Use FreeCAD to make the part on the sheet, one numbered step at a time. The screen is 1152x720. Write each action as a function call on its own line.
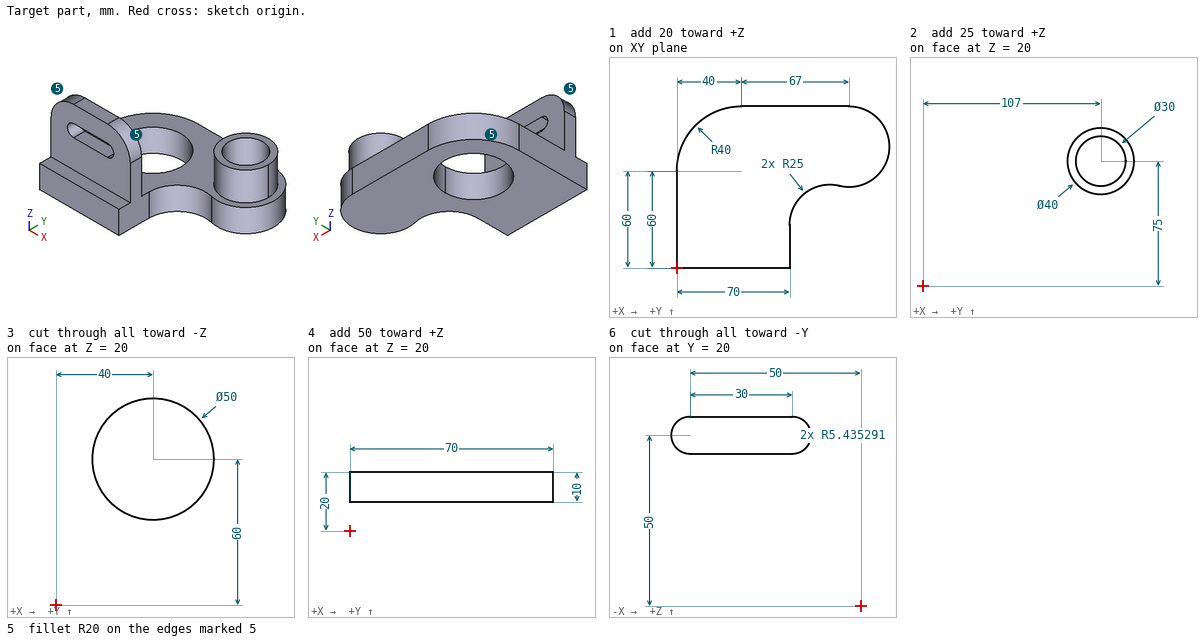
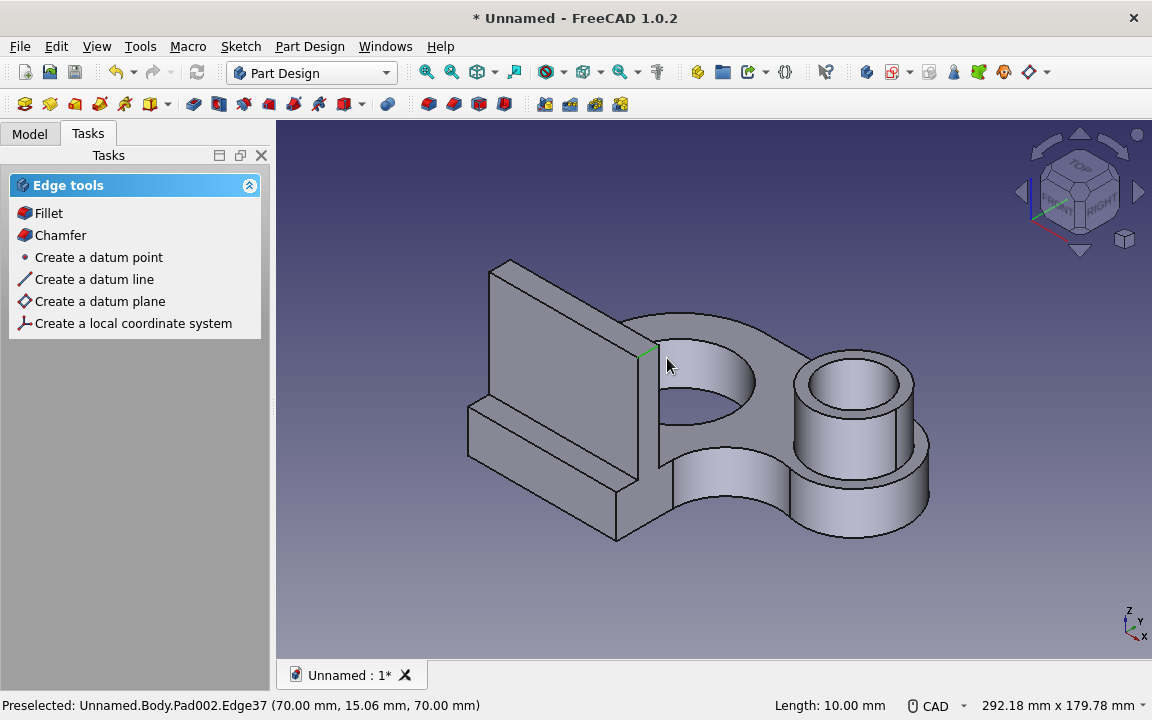
key(2)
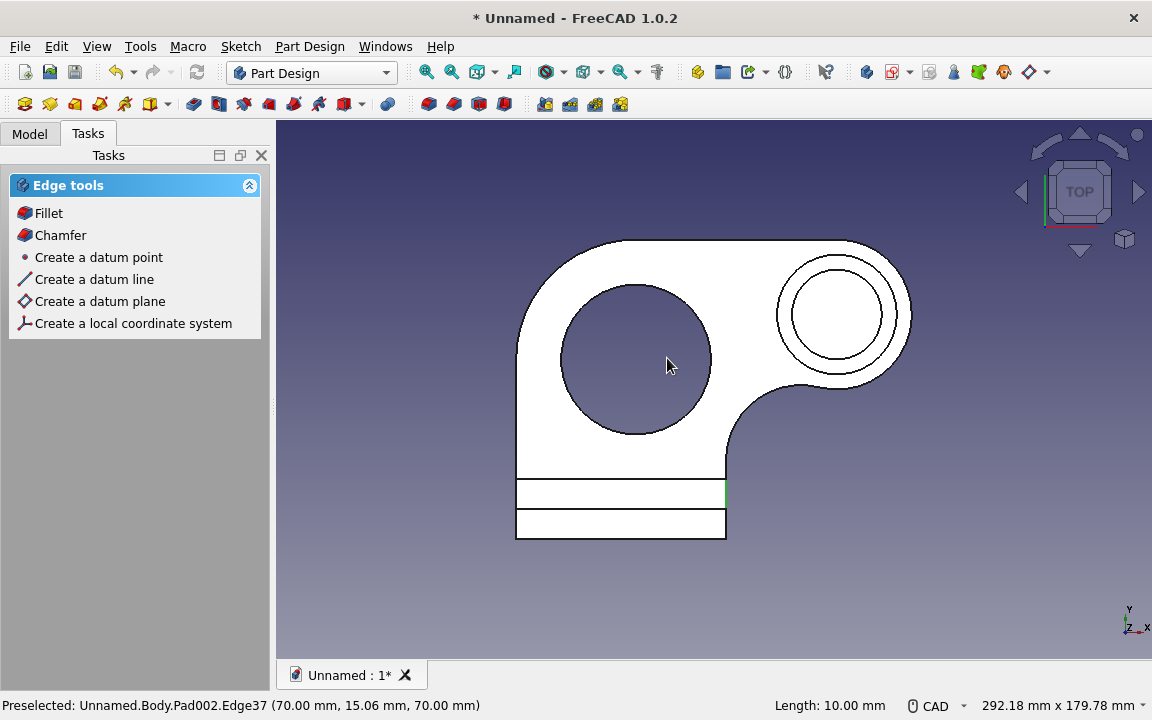
click(516, 493, ctrl)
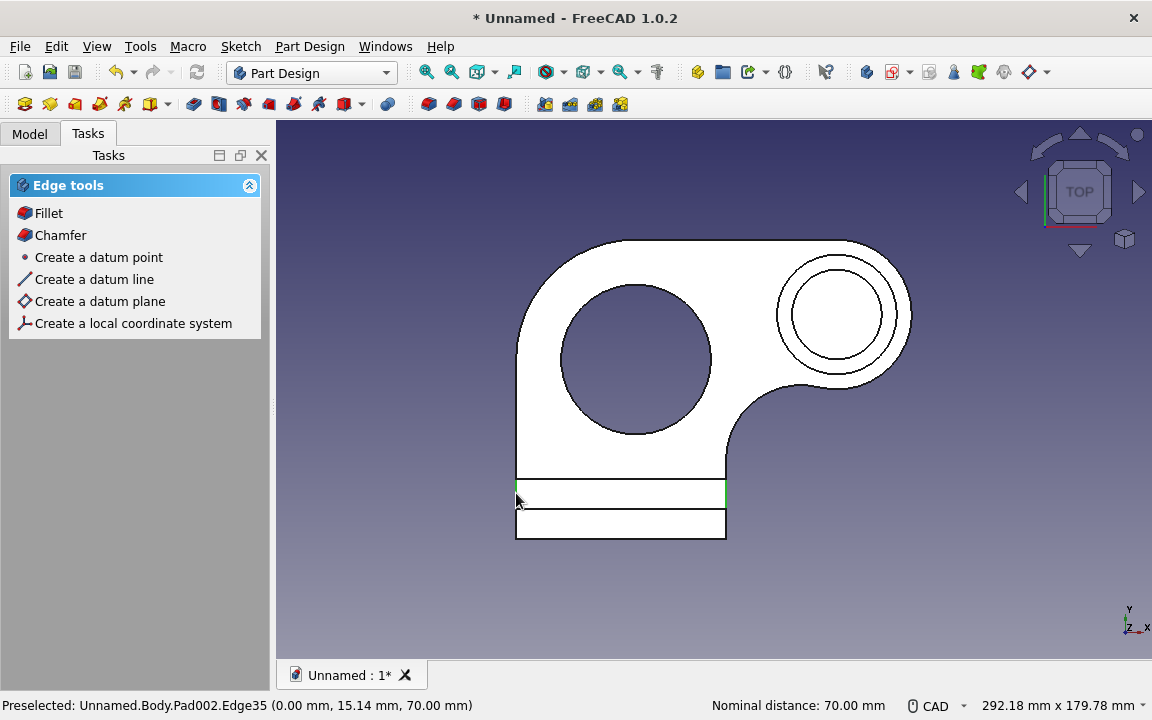
click(429, 104)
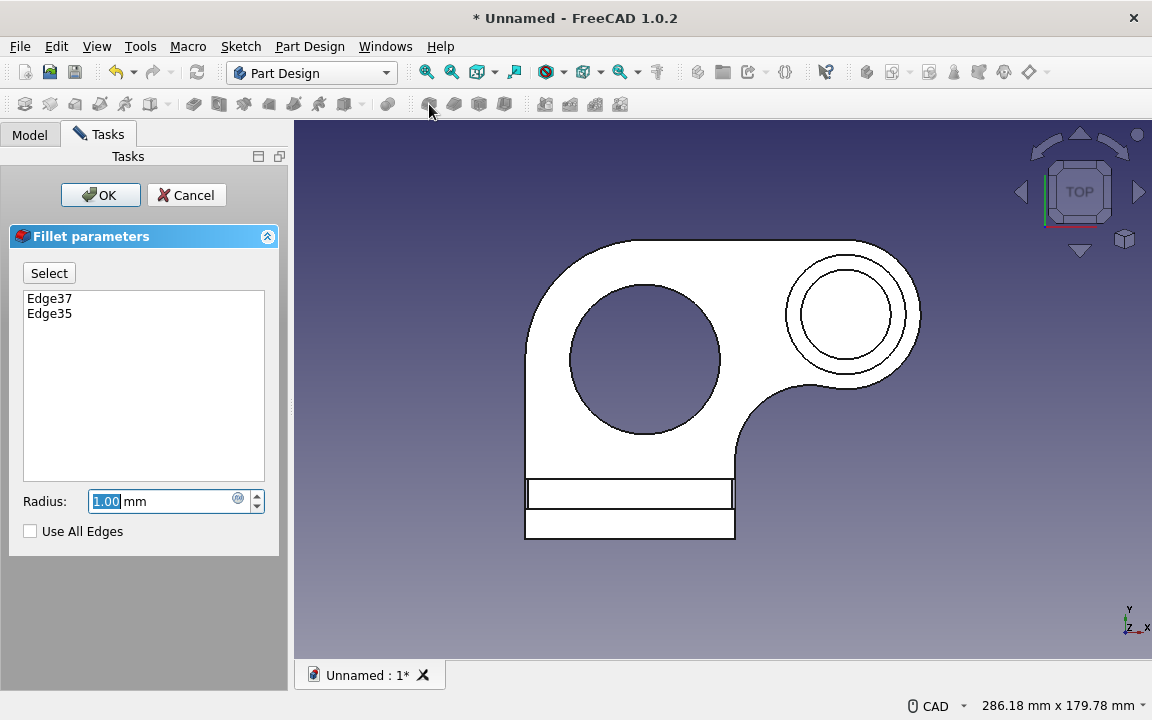
text(20)
key(Tab)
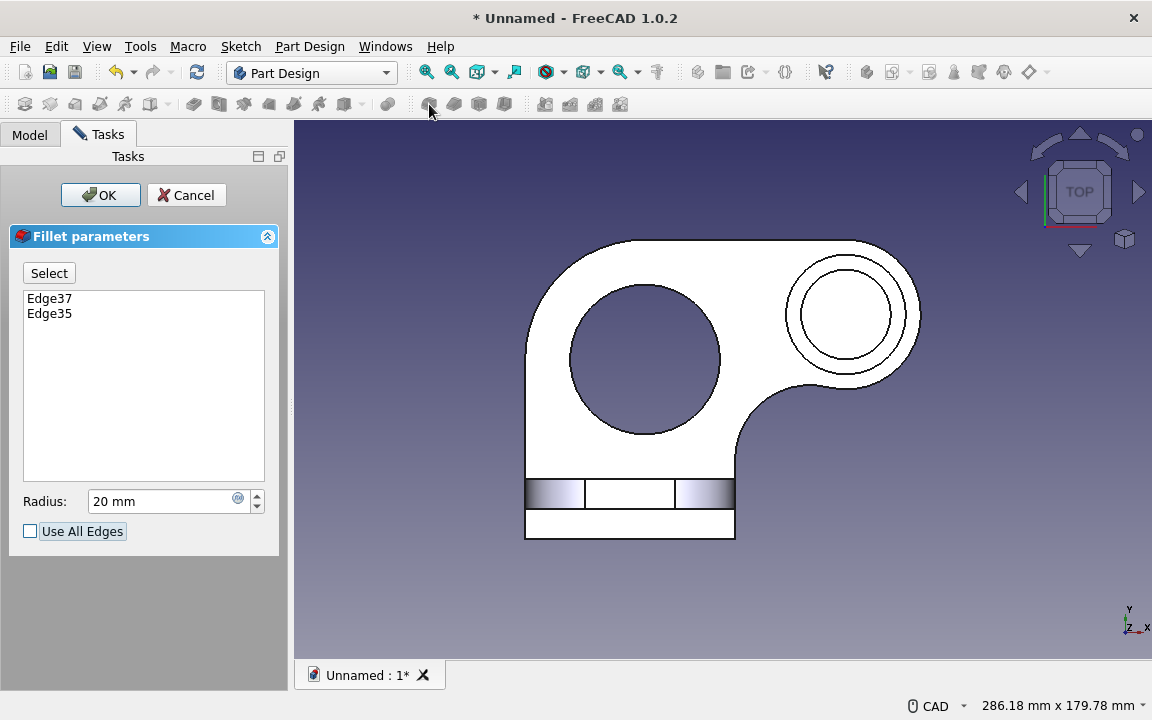
click(101, 195)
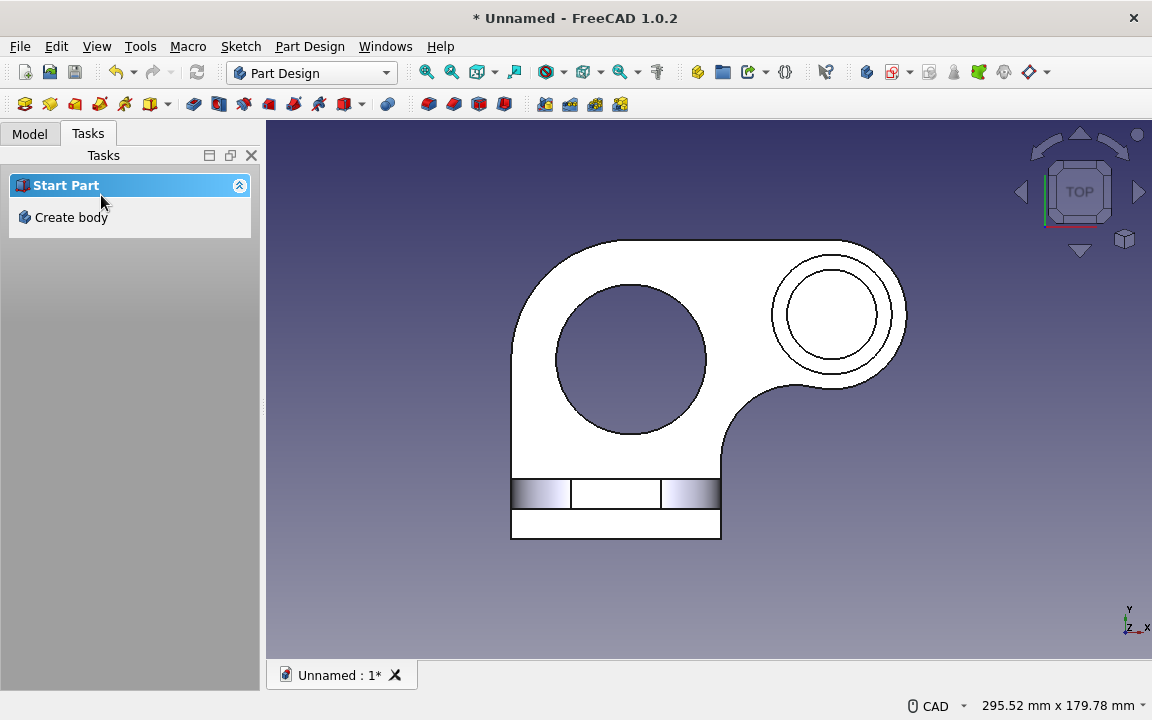
key(4)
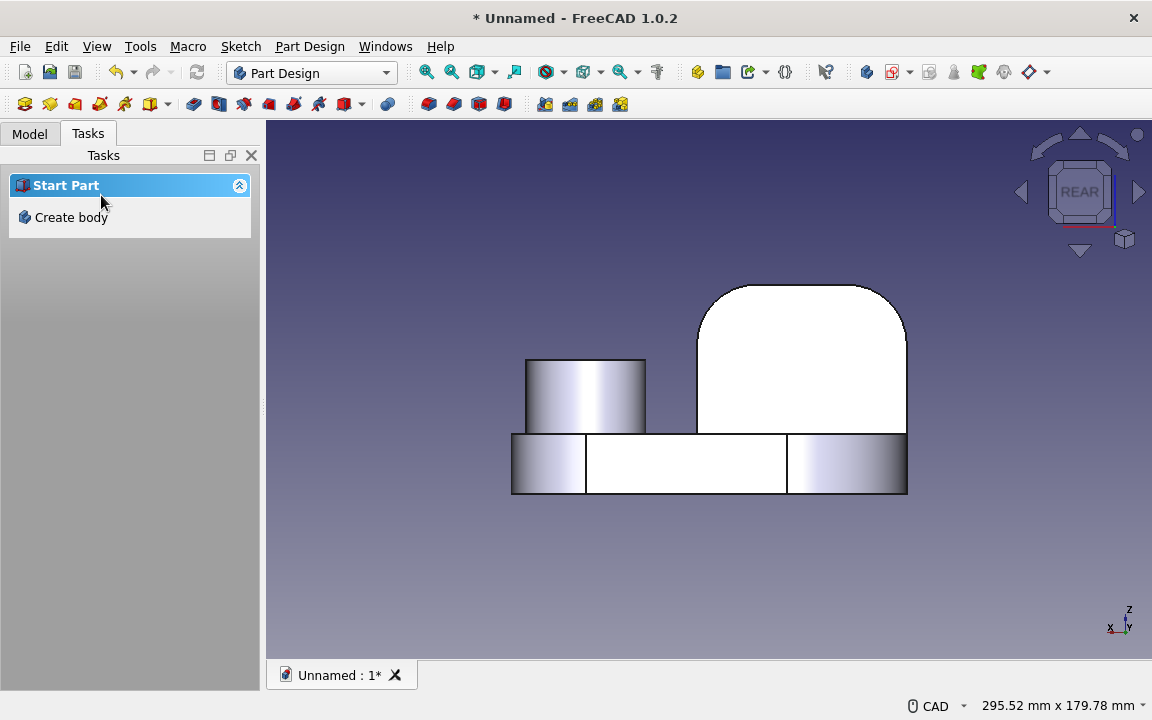
click(427, 72)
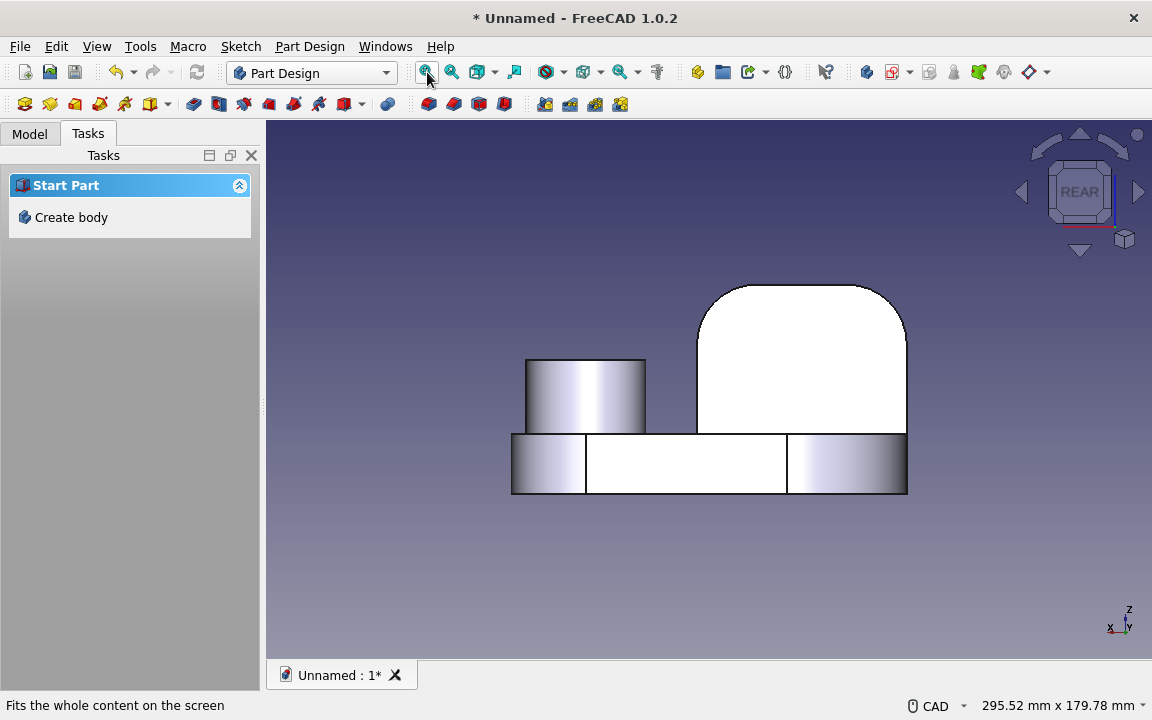
click(772, 359)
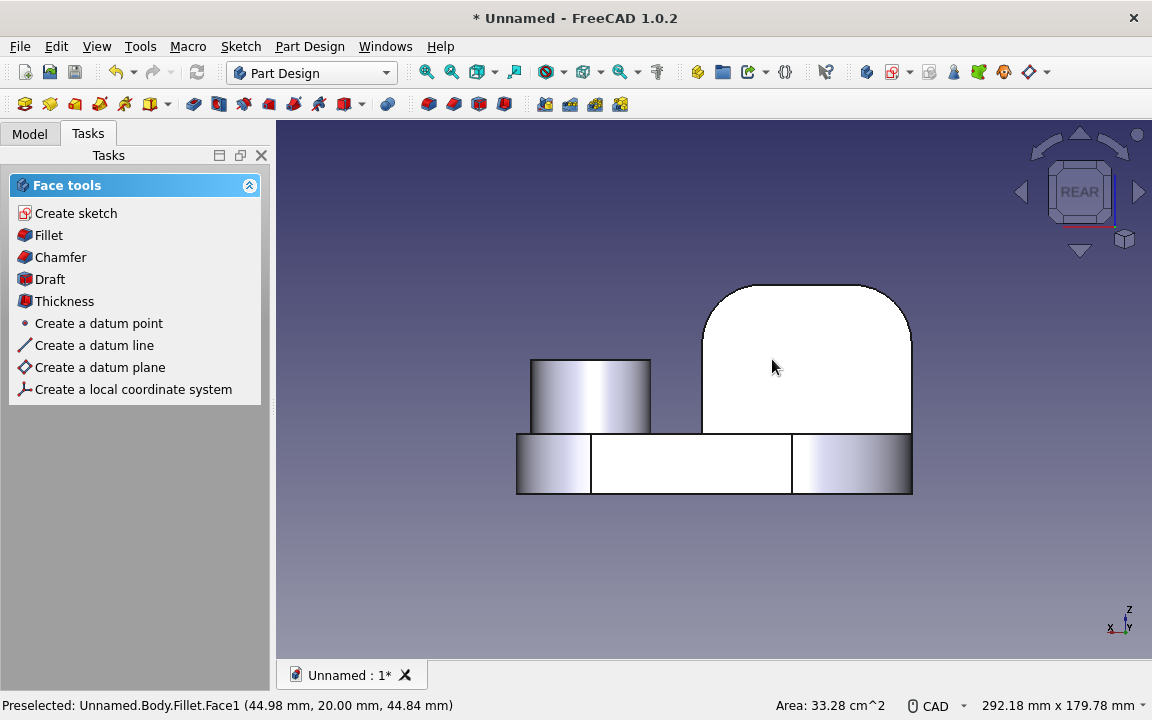
click(892, 72)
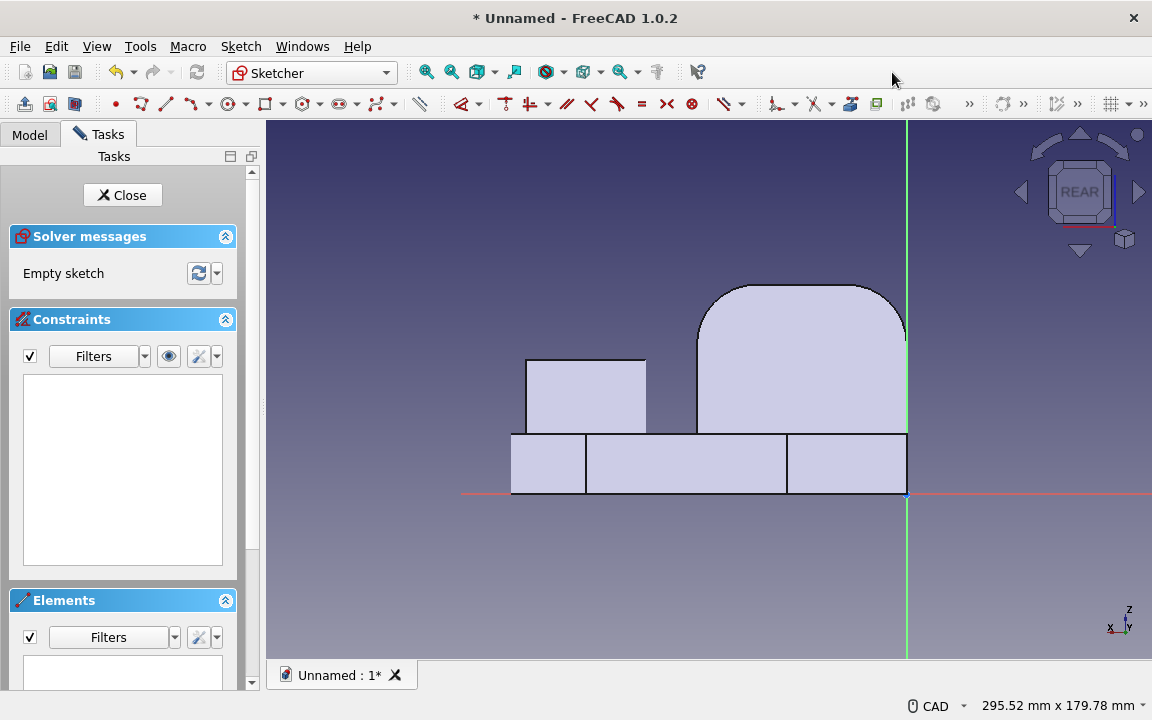
scroll(973, 429, up, 4)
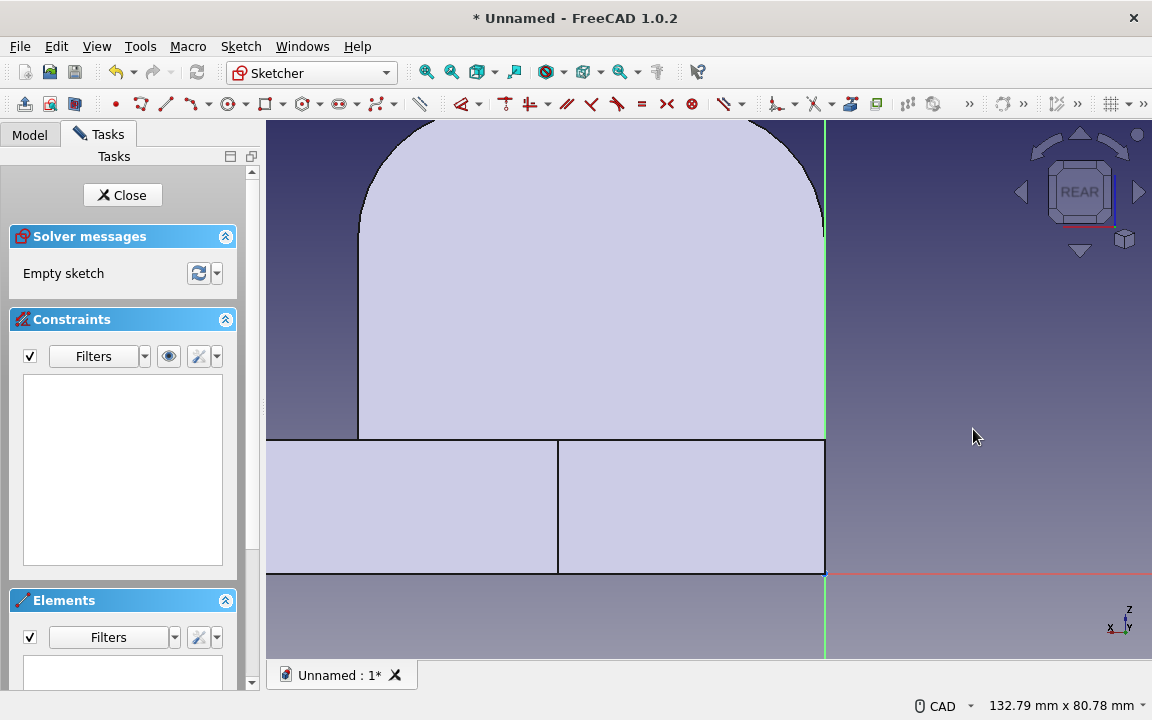
click(338, 104)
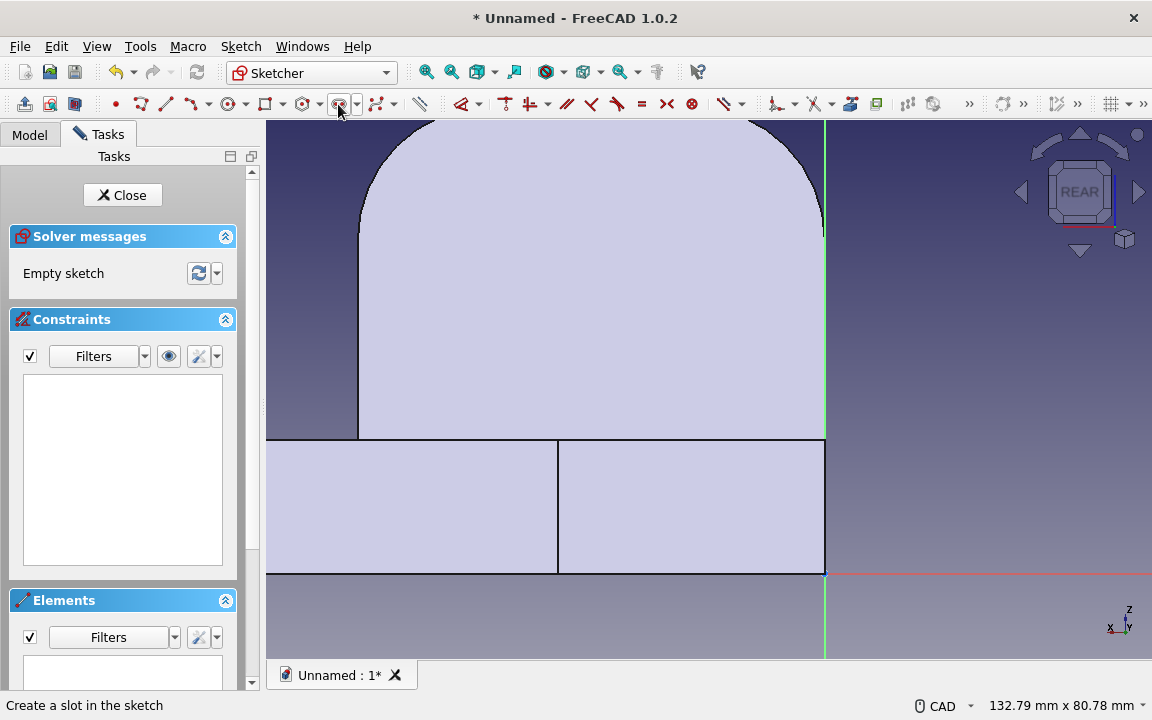
click(491, 240)